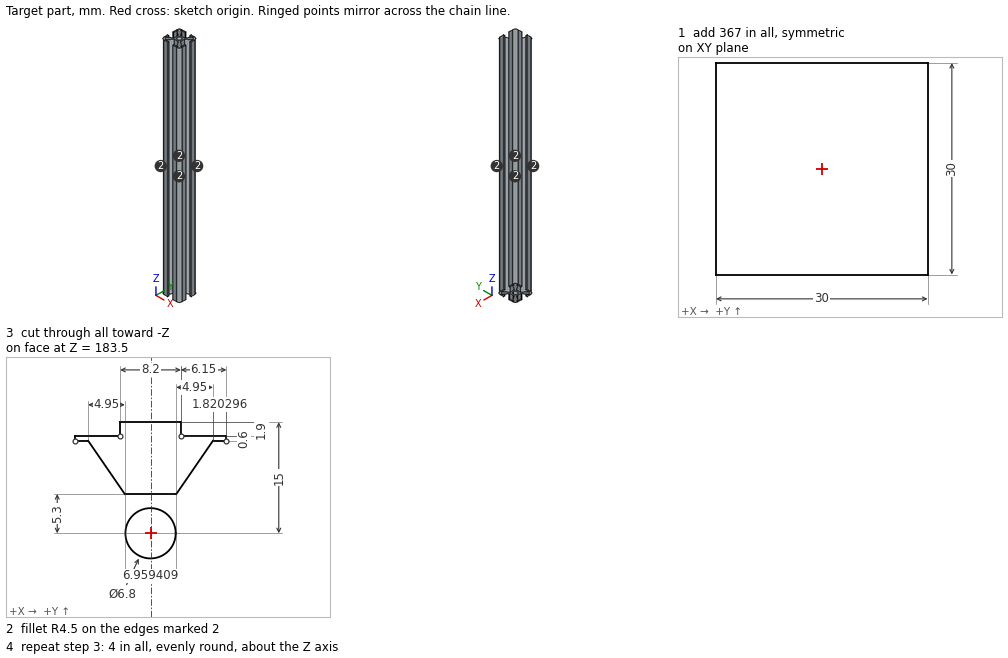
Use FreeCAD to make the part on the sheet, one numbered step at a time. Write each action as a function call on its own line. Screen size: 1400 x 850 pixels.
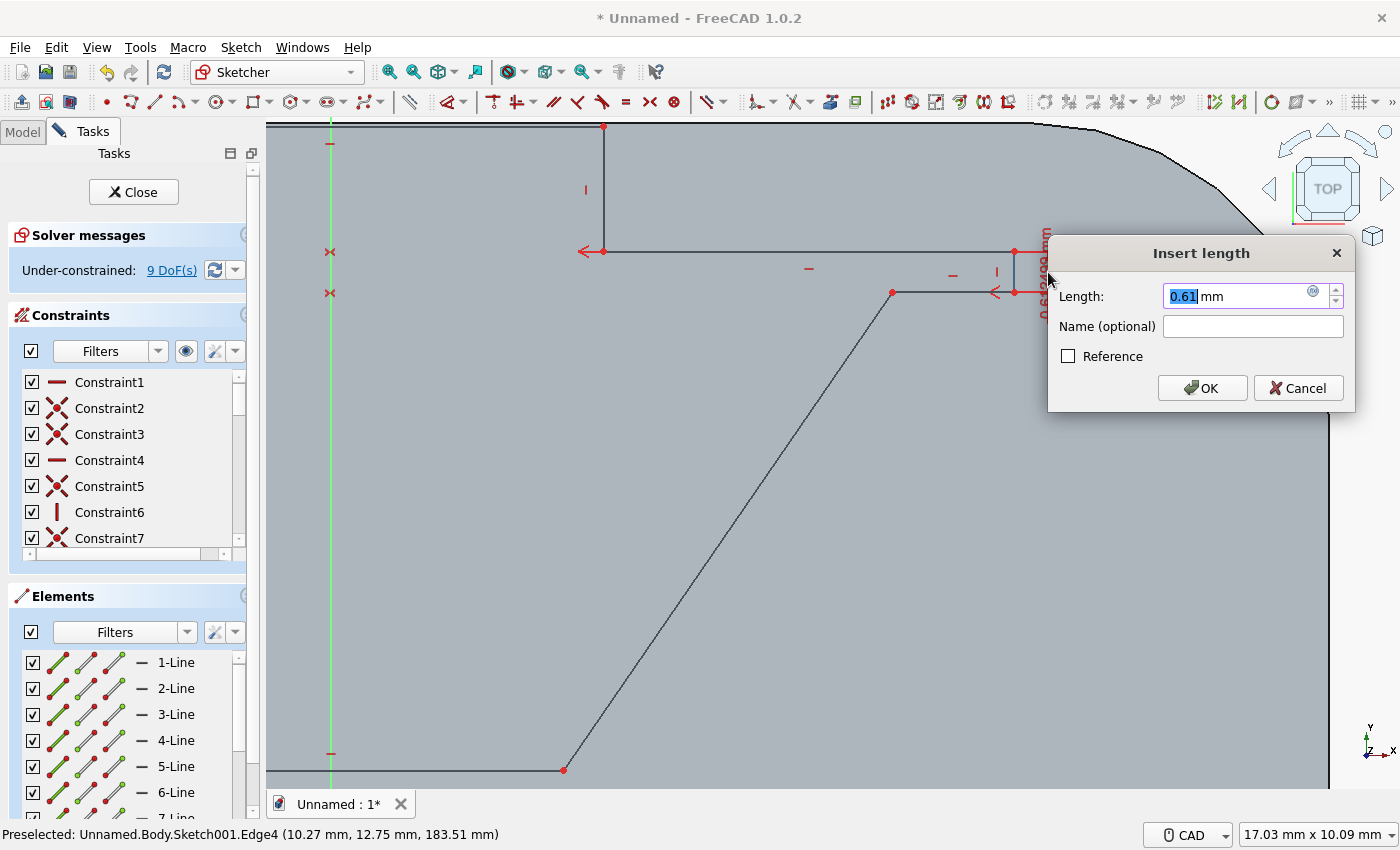
text(0.6)
key(Return)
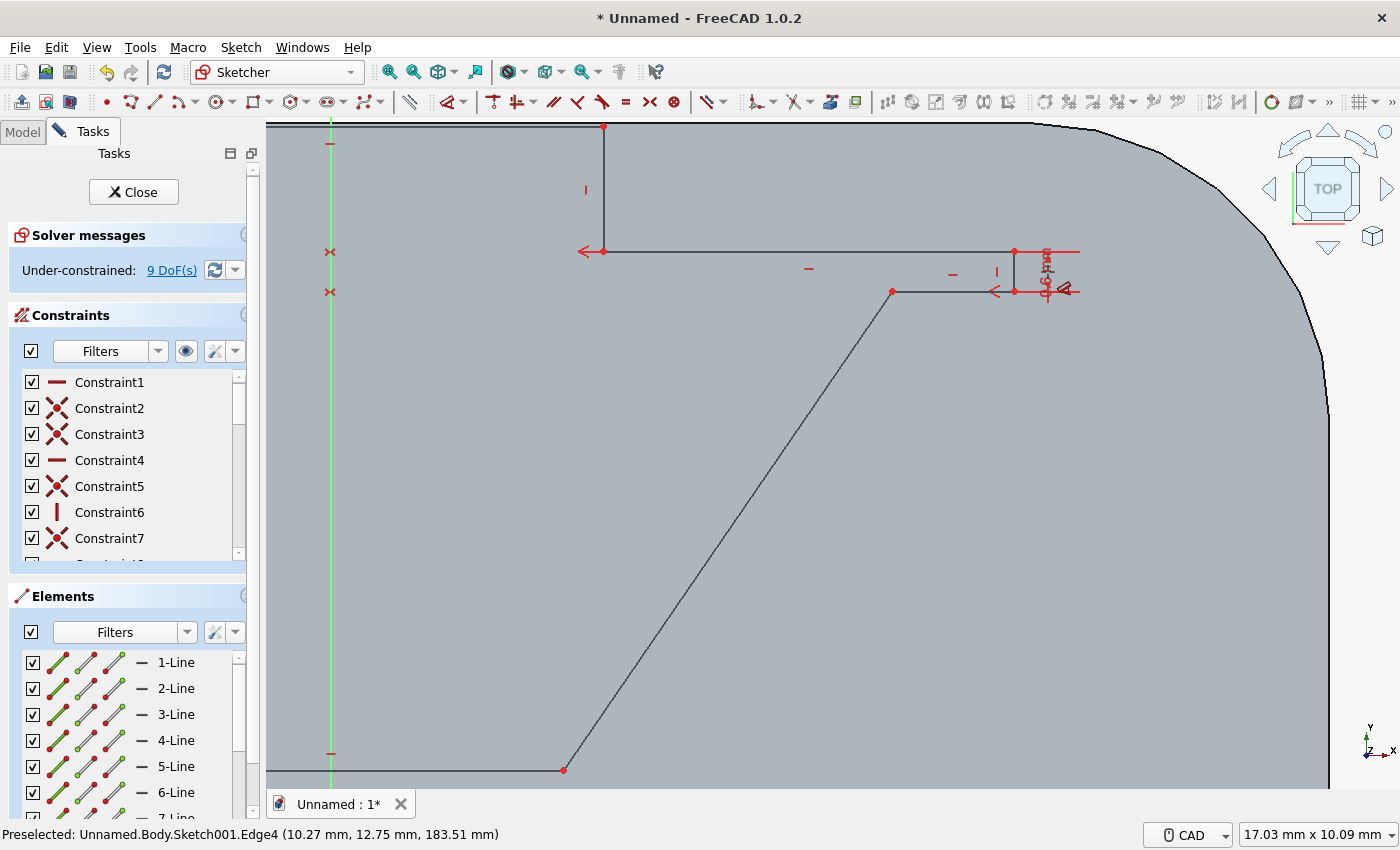
click(604, 214)
click(638, 198)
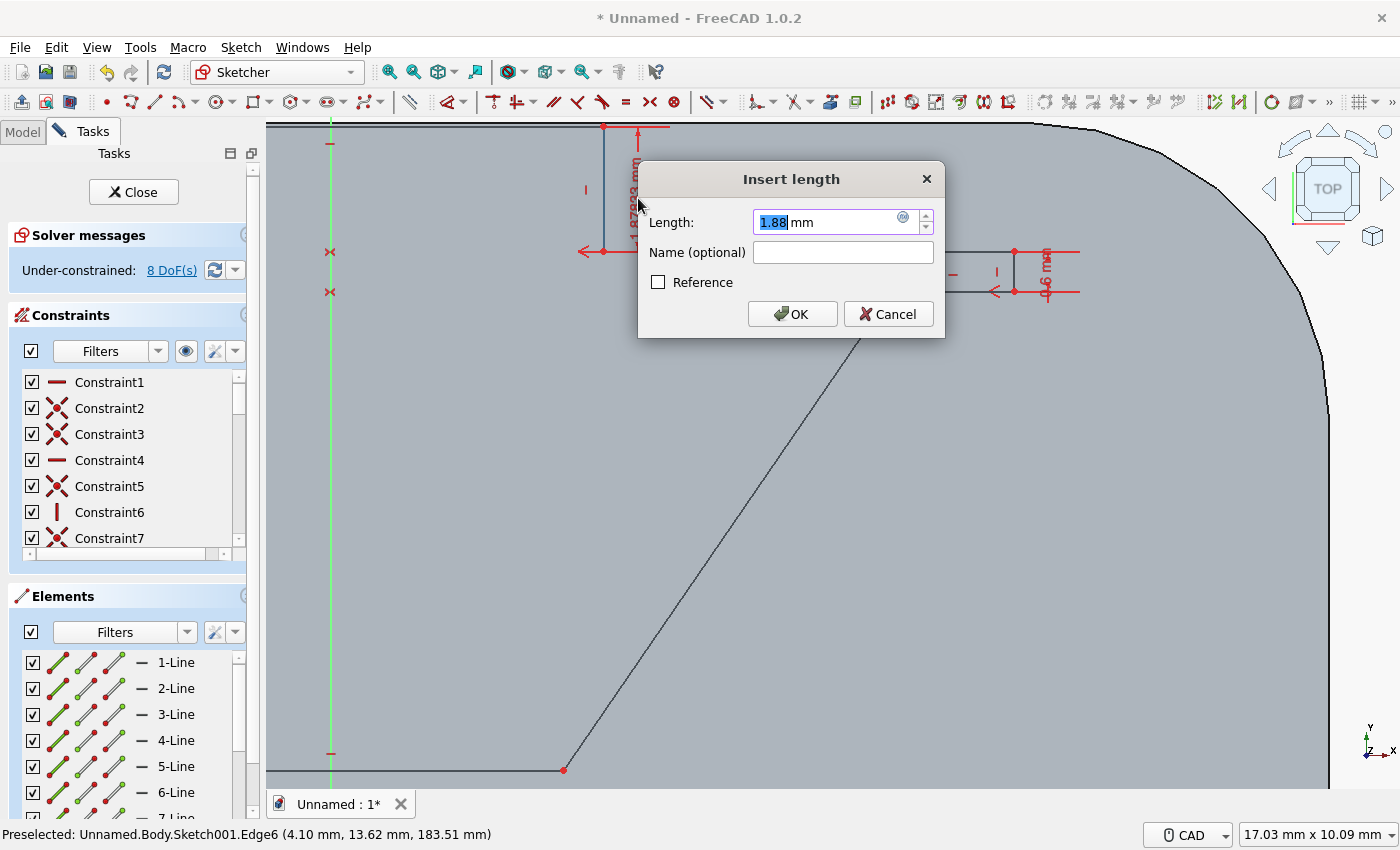
text(1.9)
key(Return)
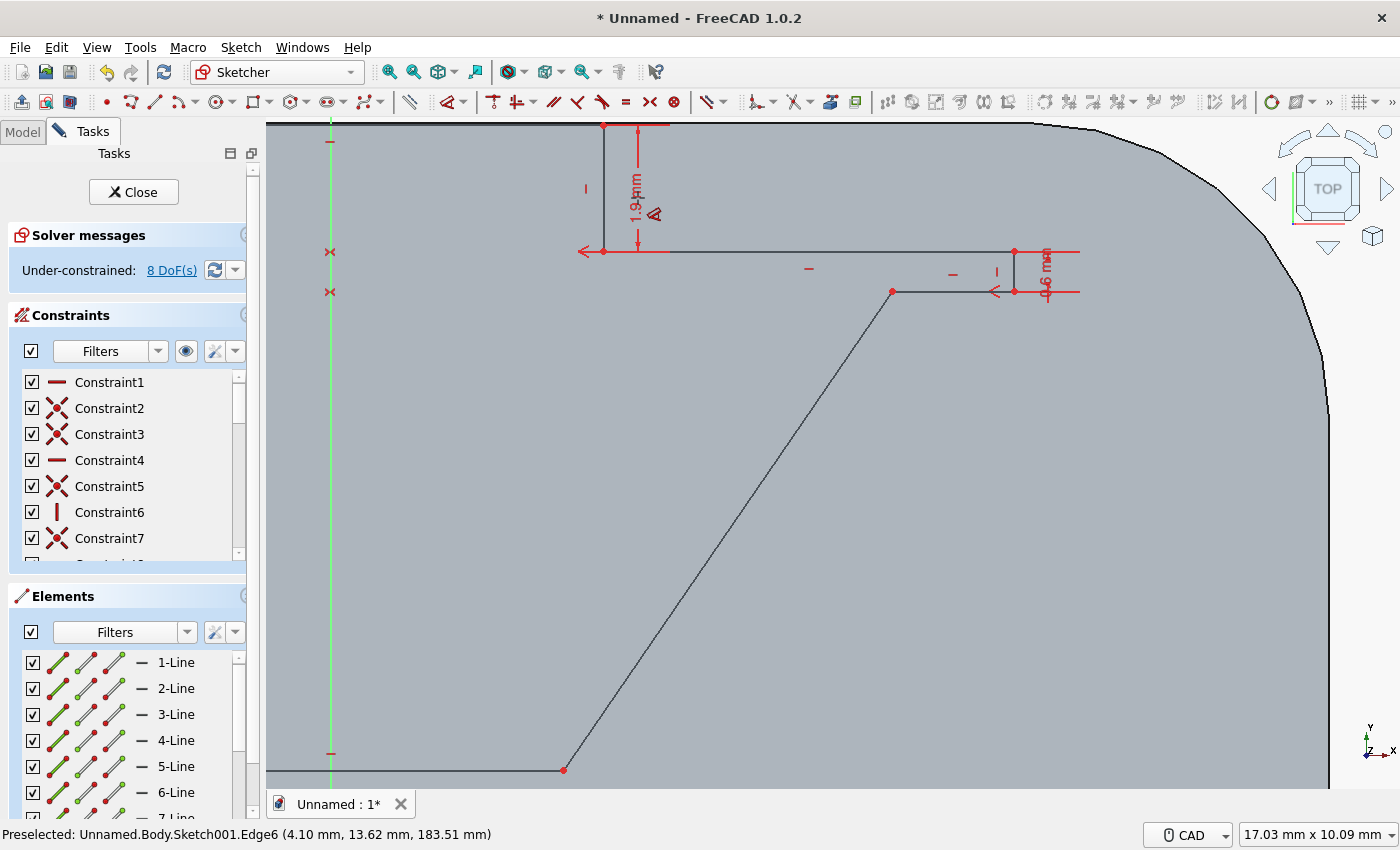
scroll(1017, 289, down, 5)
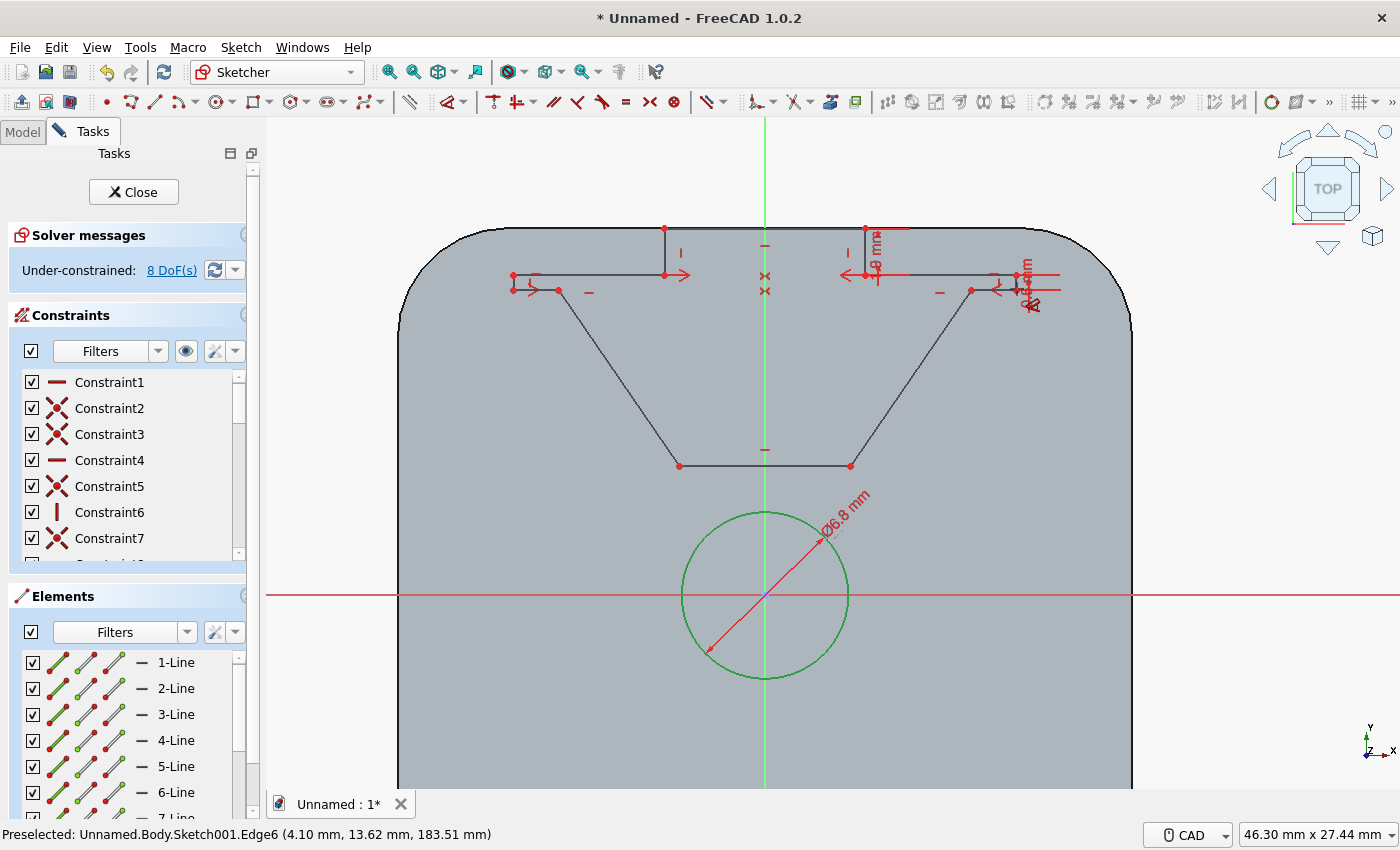
click(805, 229)
click(719, 195)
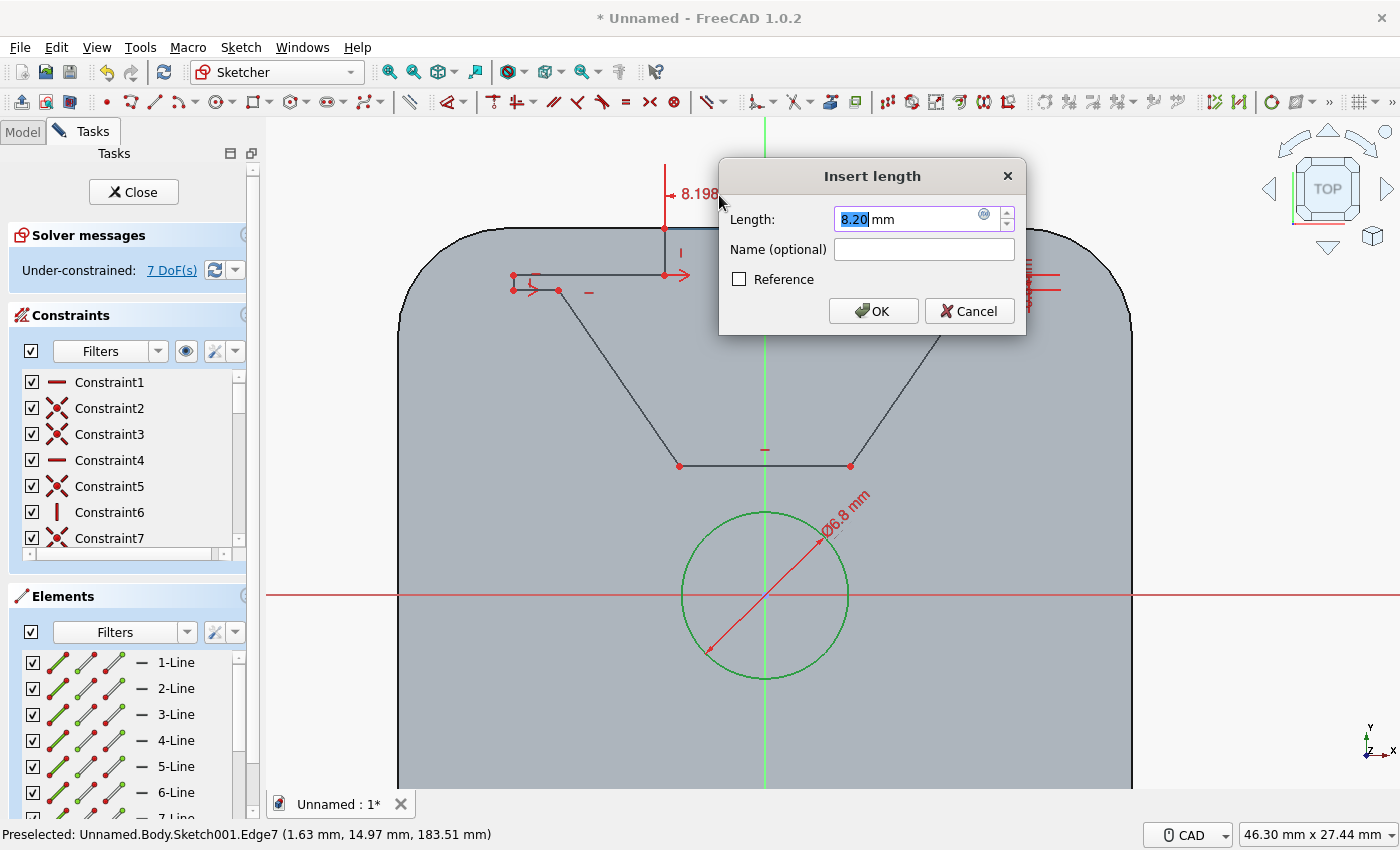
text(8.2)
key(Return)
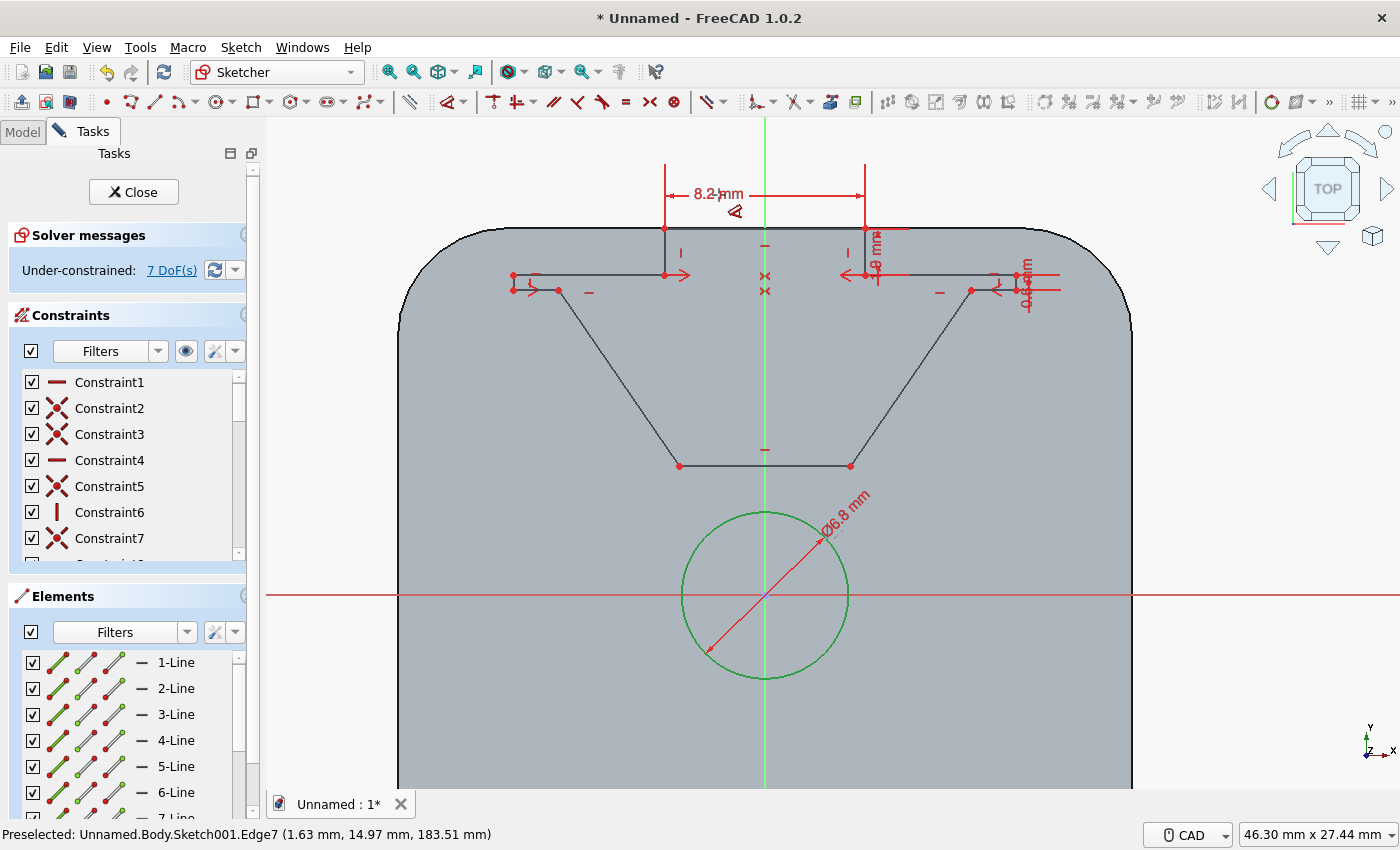
click(865, 229)
click(899, 328)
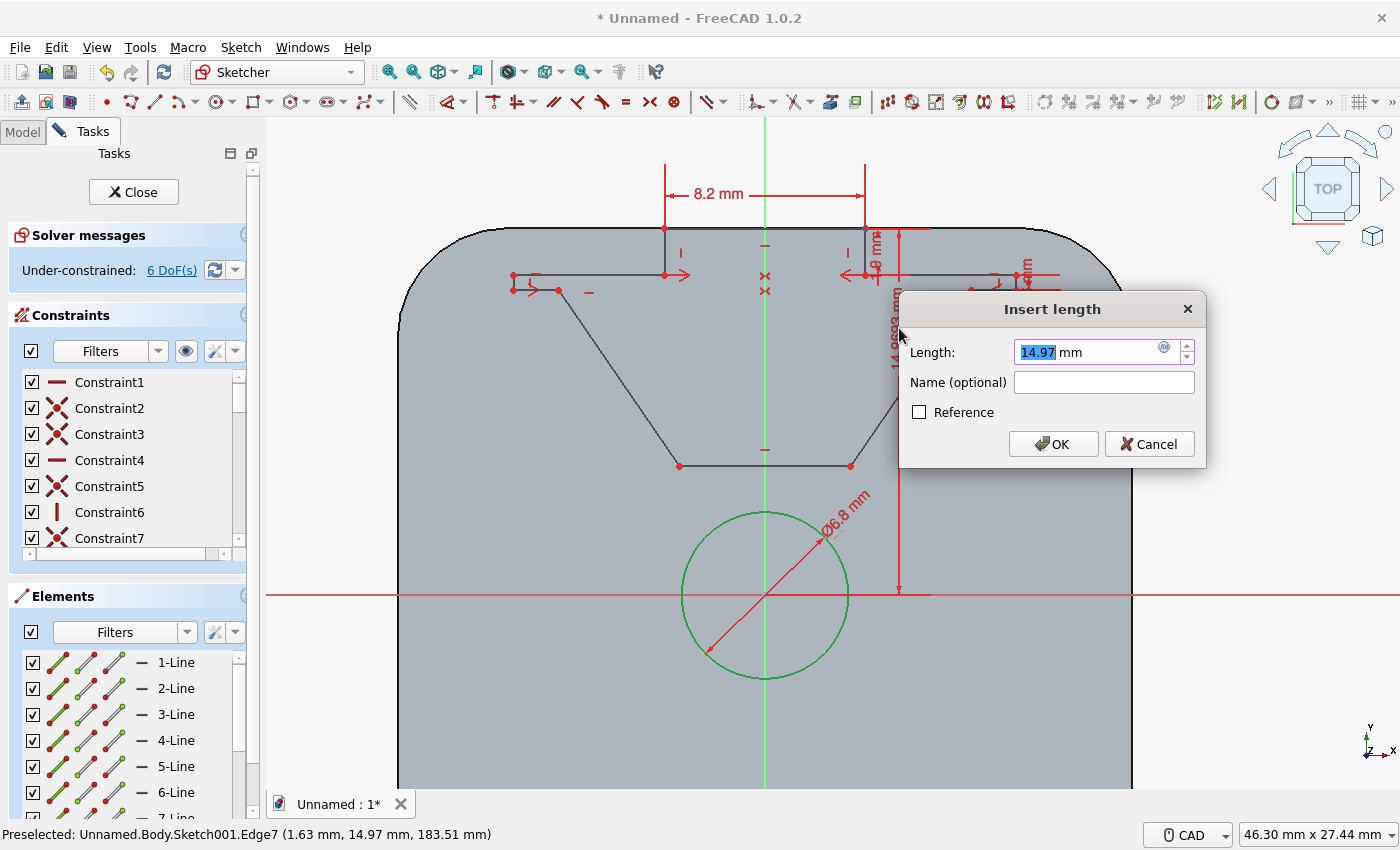
text(15)
key(Return)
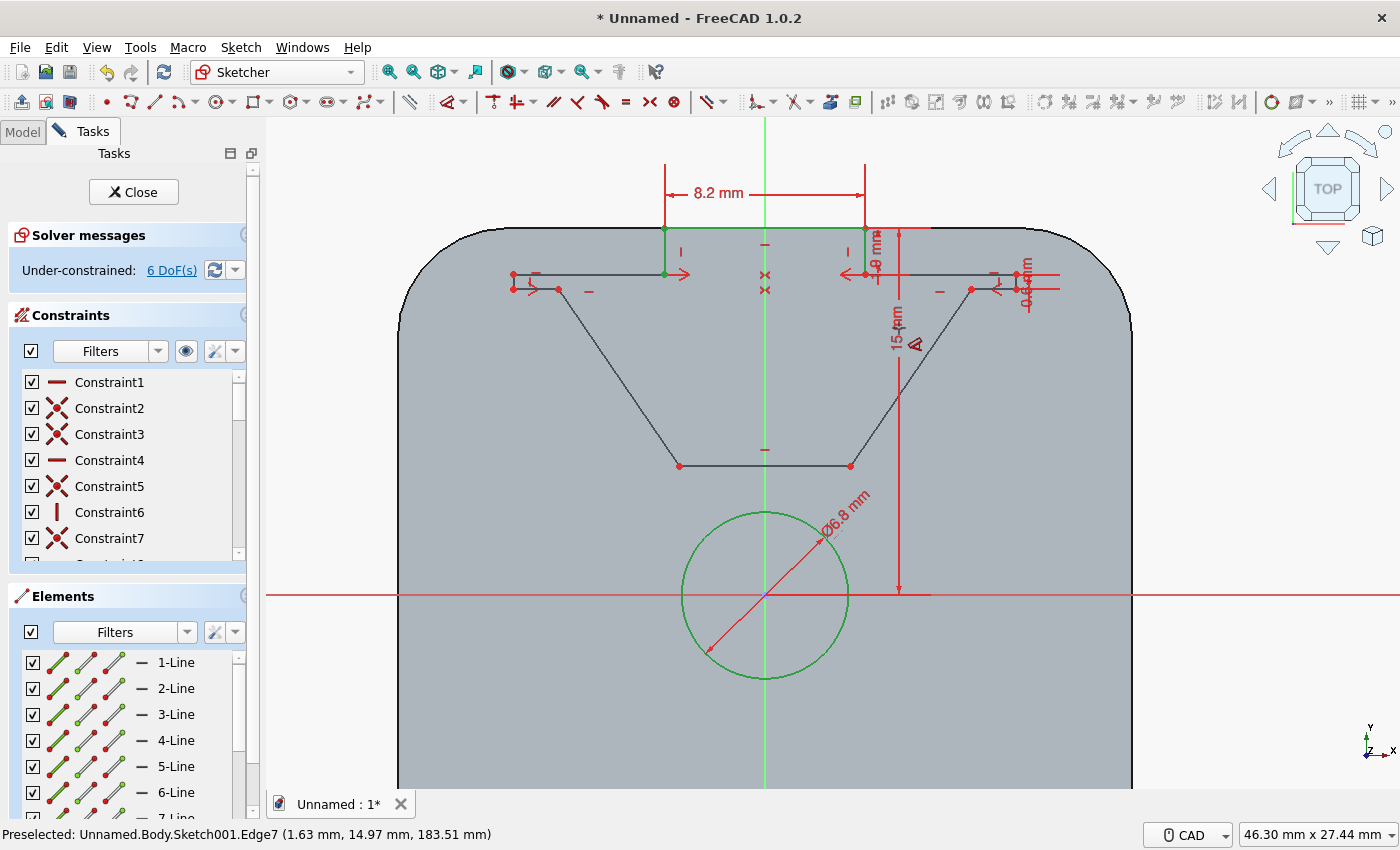
click(971, 275)
click(976, 241)